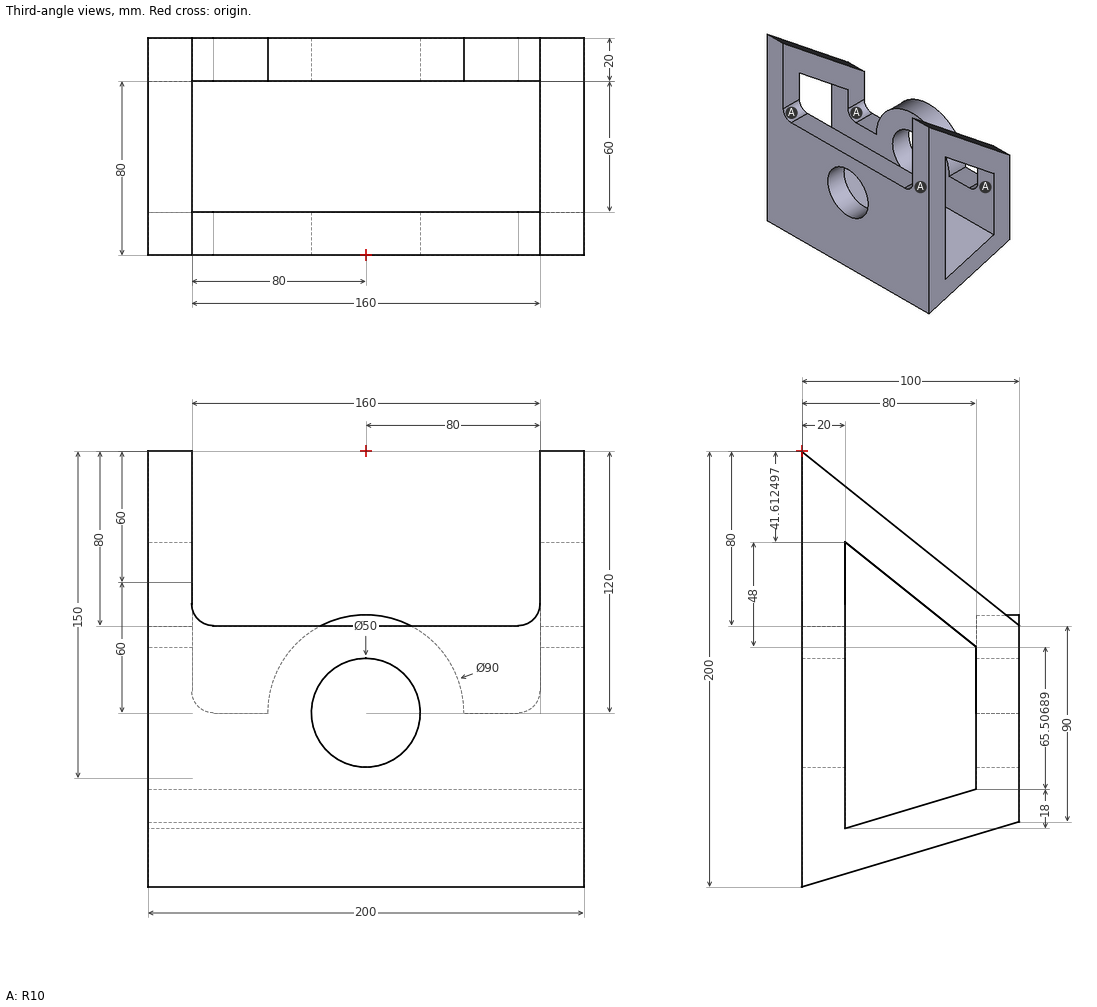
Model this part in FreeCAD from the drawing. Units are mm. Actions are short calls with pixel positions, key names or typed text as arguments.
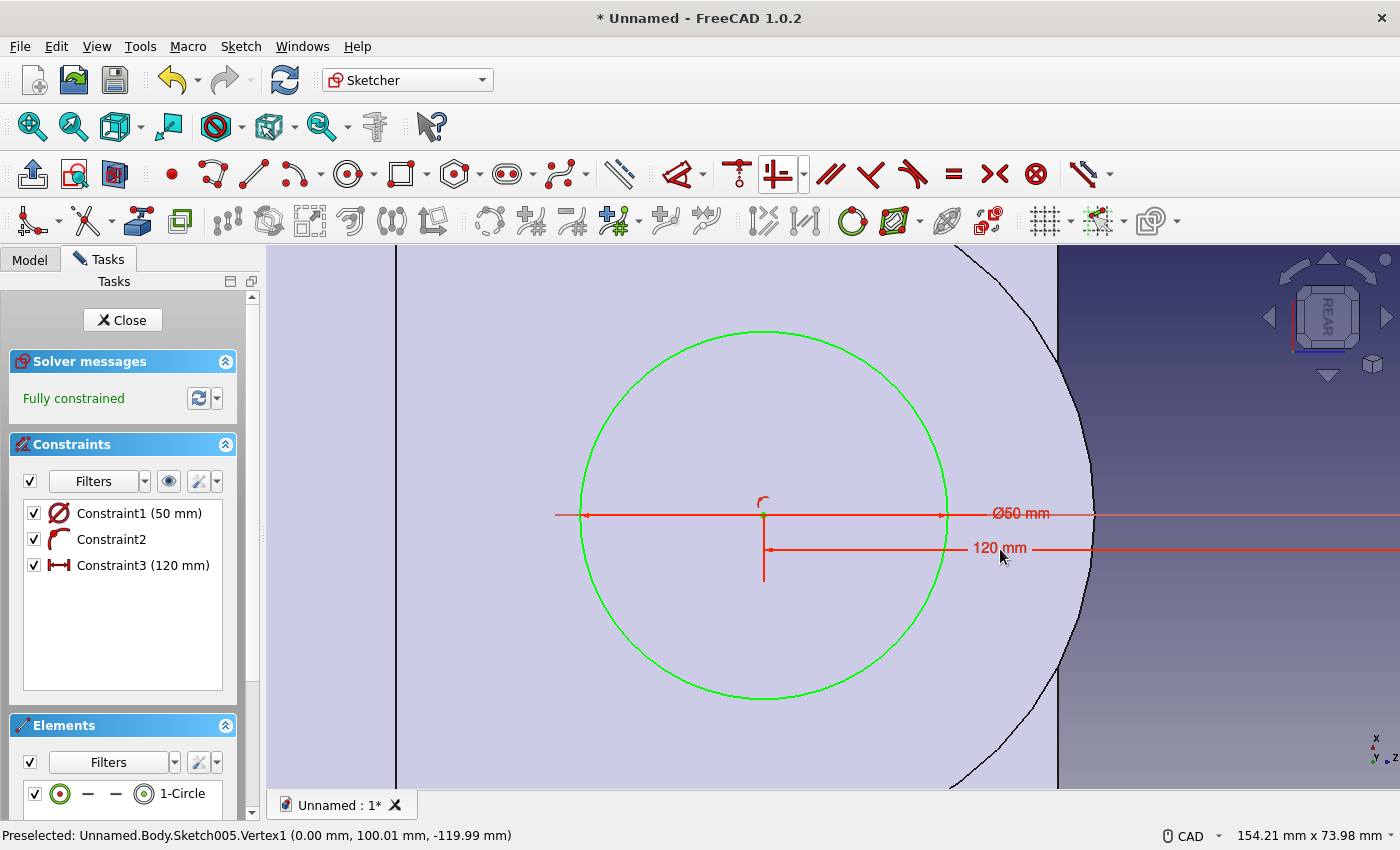
click(123, 320)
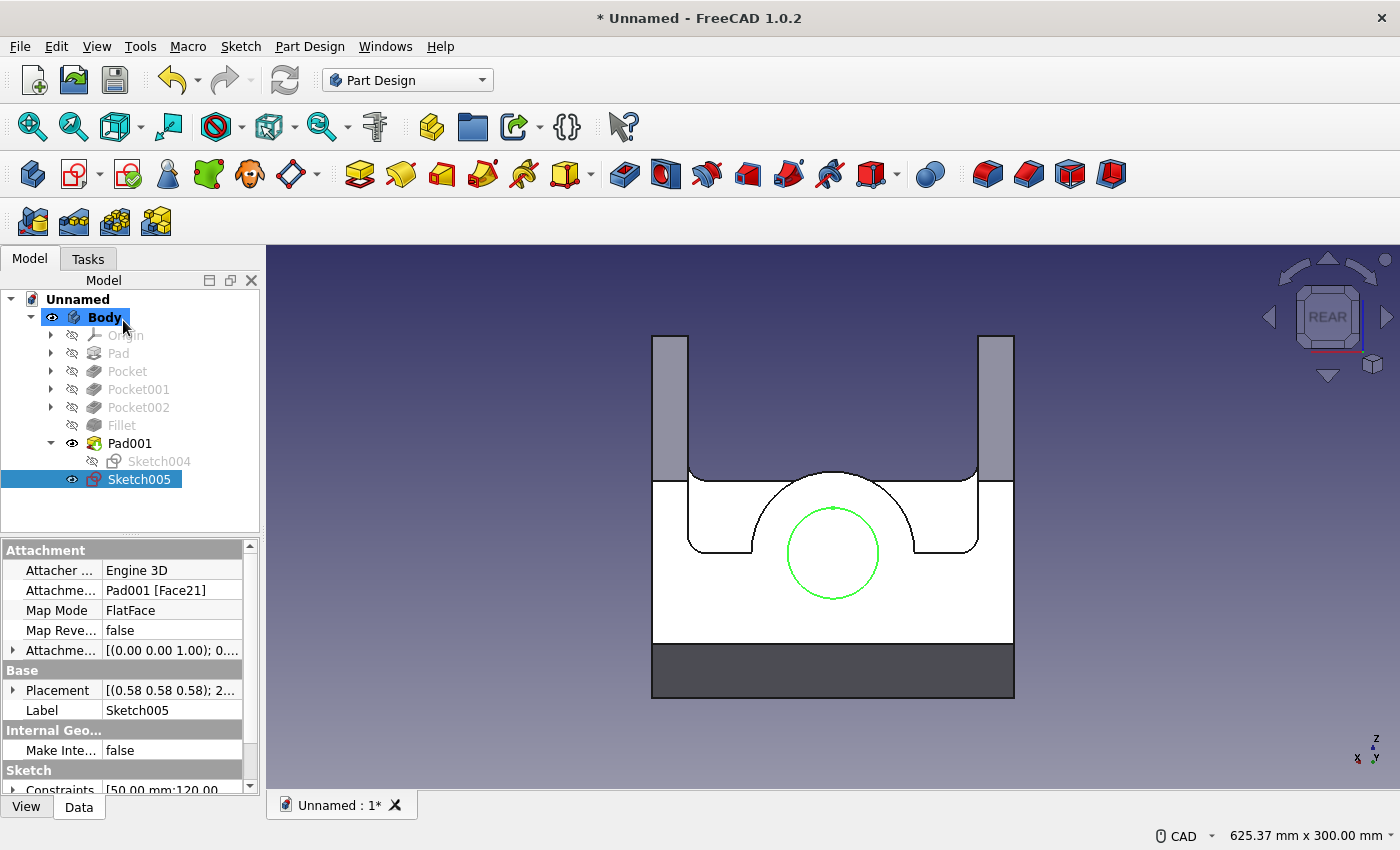
click(625, 174)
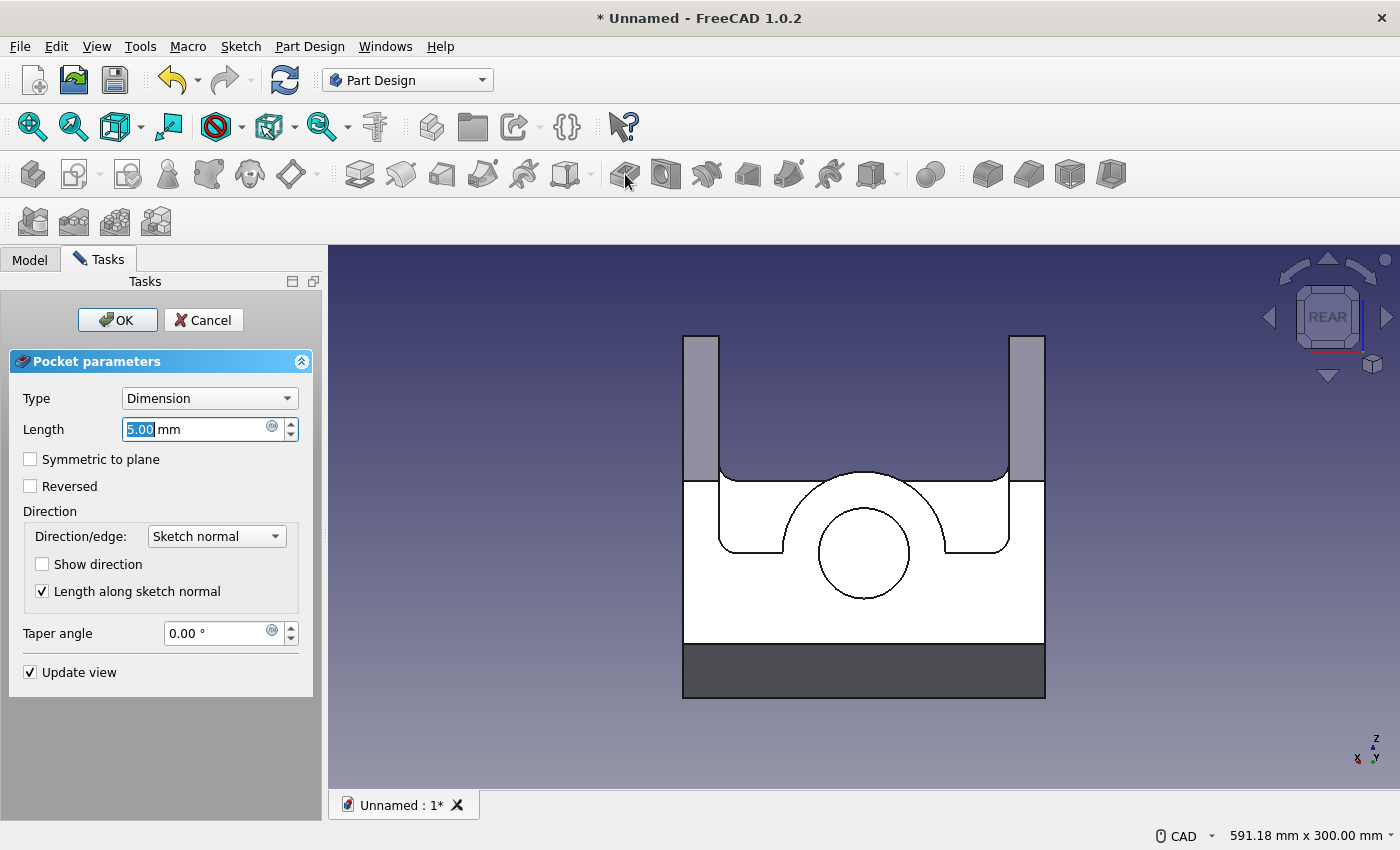
click(210, 398)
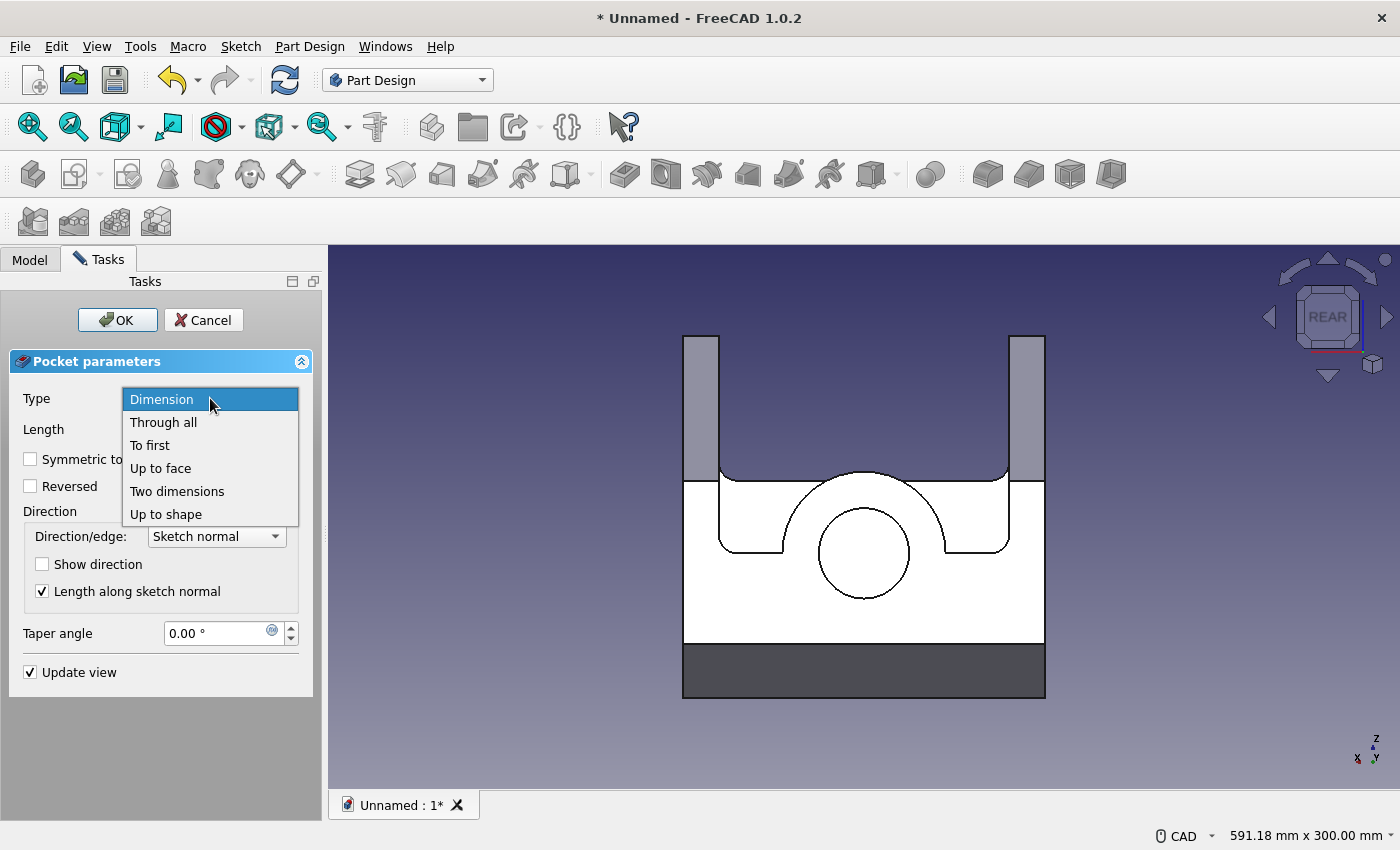
click(208, 422)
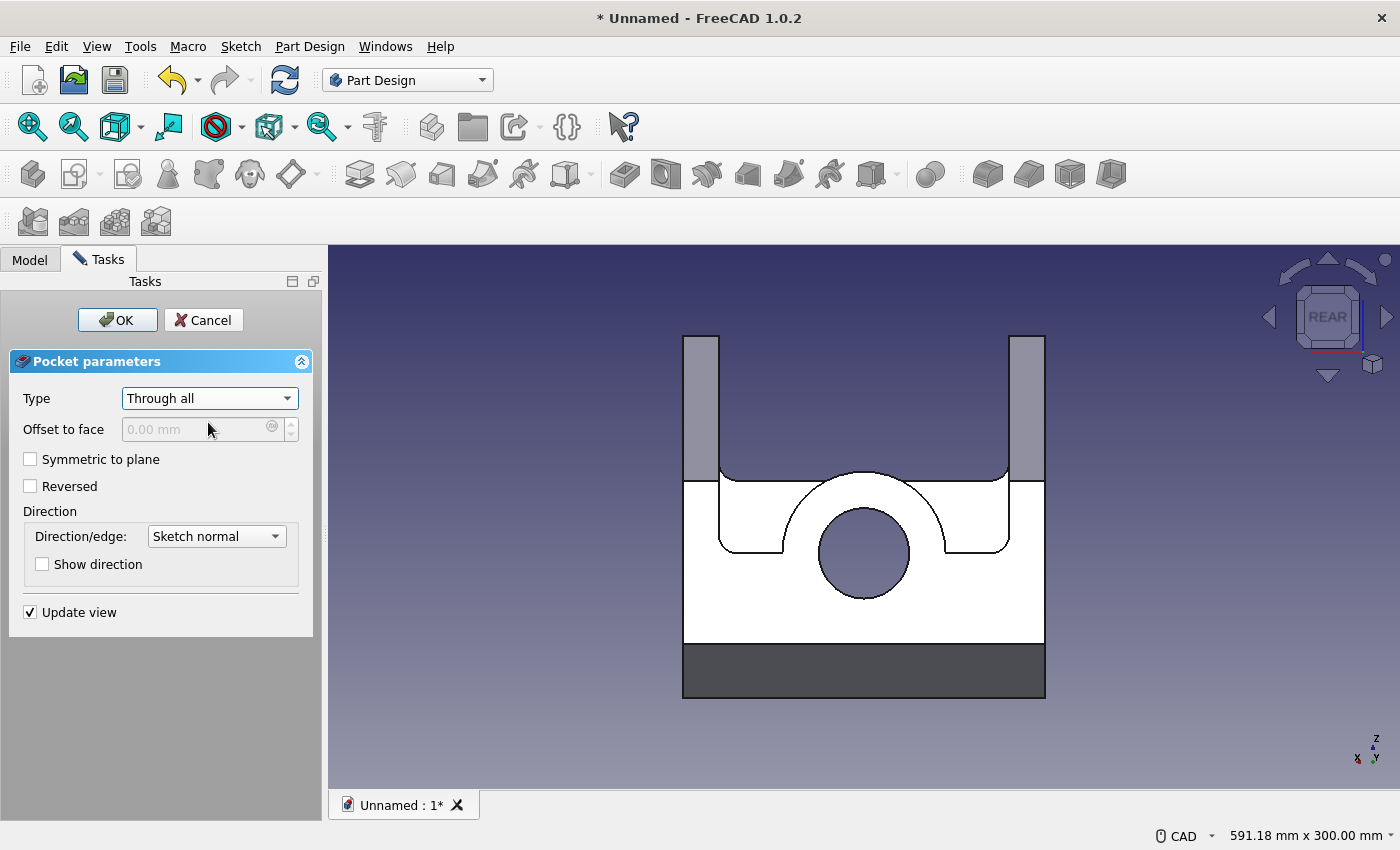
click(118, 320)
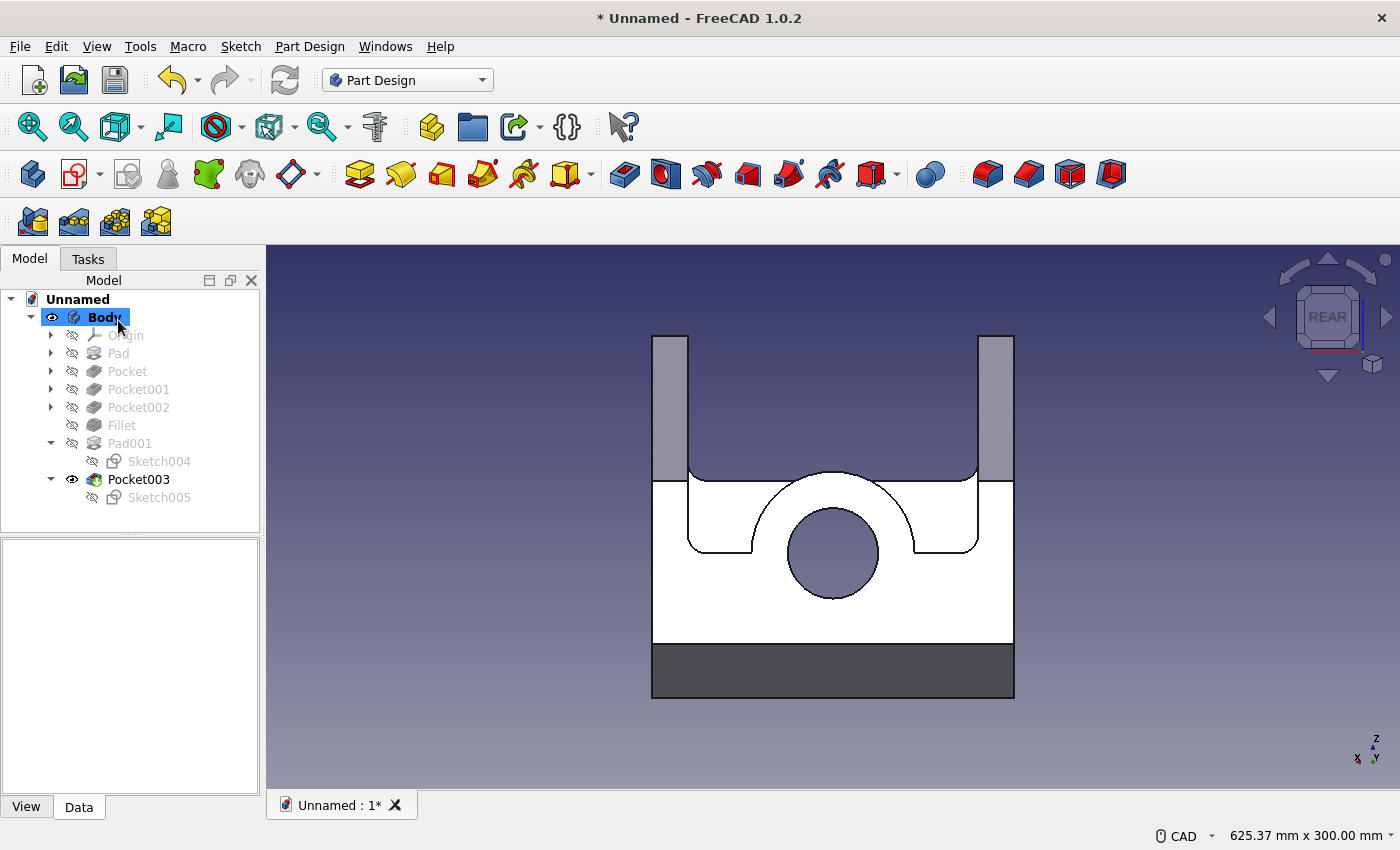
key(0)